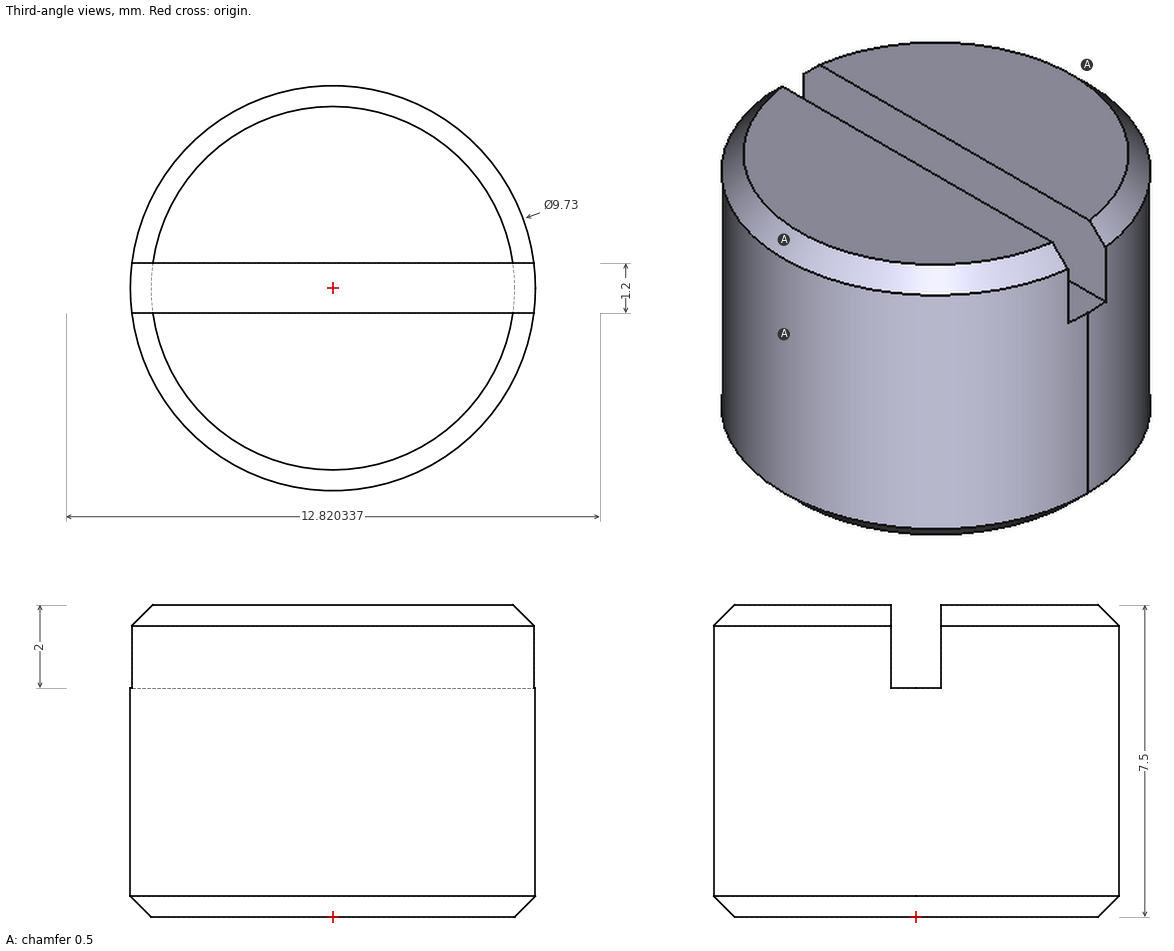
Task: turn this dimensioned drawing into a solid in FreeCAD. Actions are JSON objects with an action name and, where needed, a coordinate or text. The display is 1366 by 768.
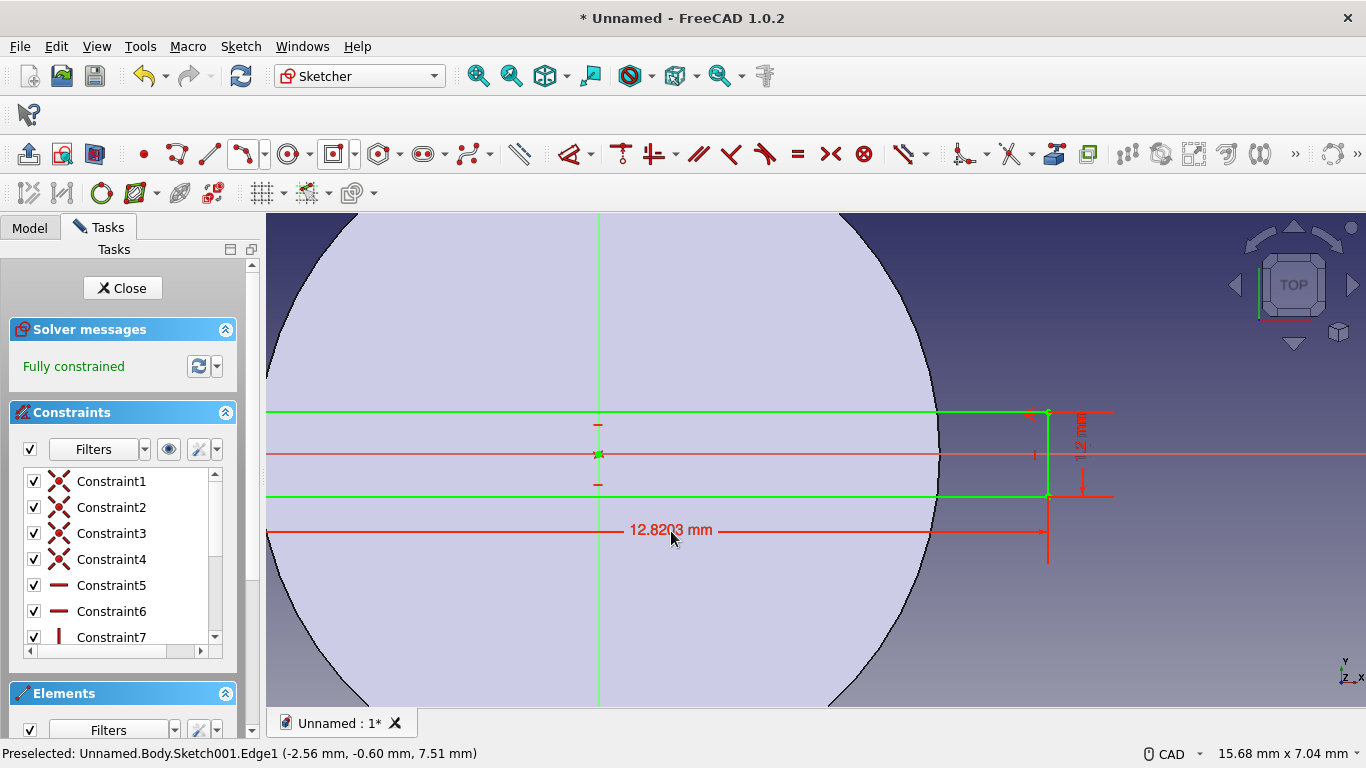
{"action": "left_click", "coordinate": [123, 288]}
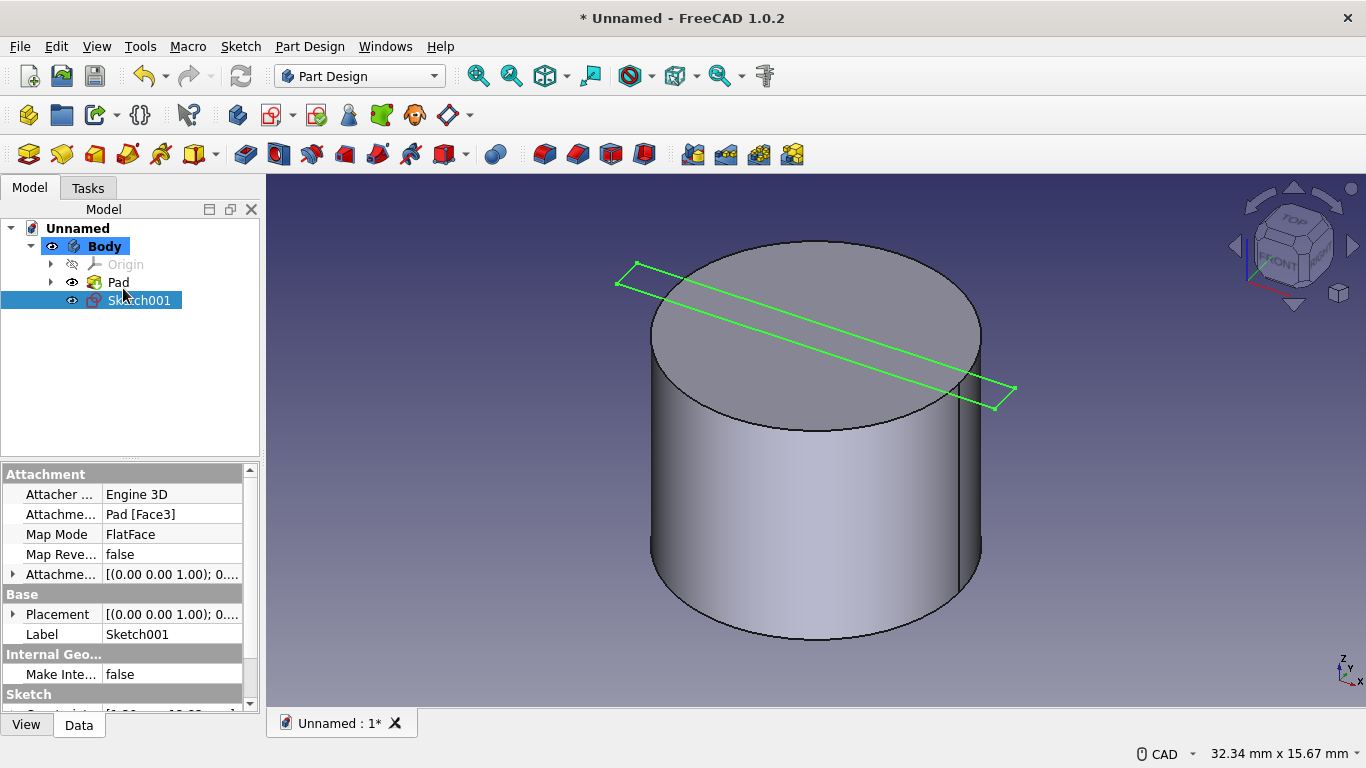
{"action": "left_click", "coordinate": [246, 154]}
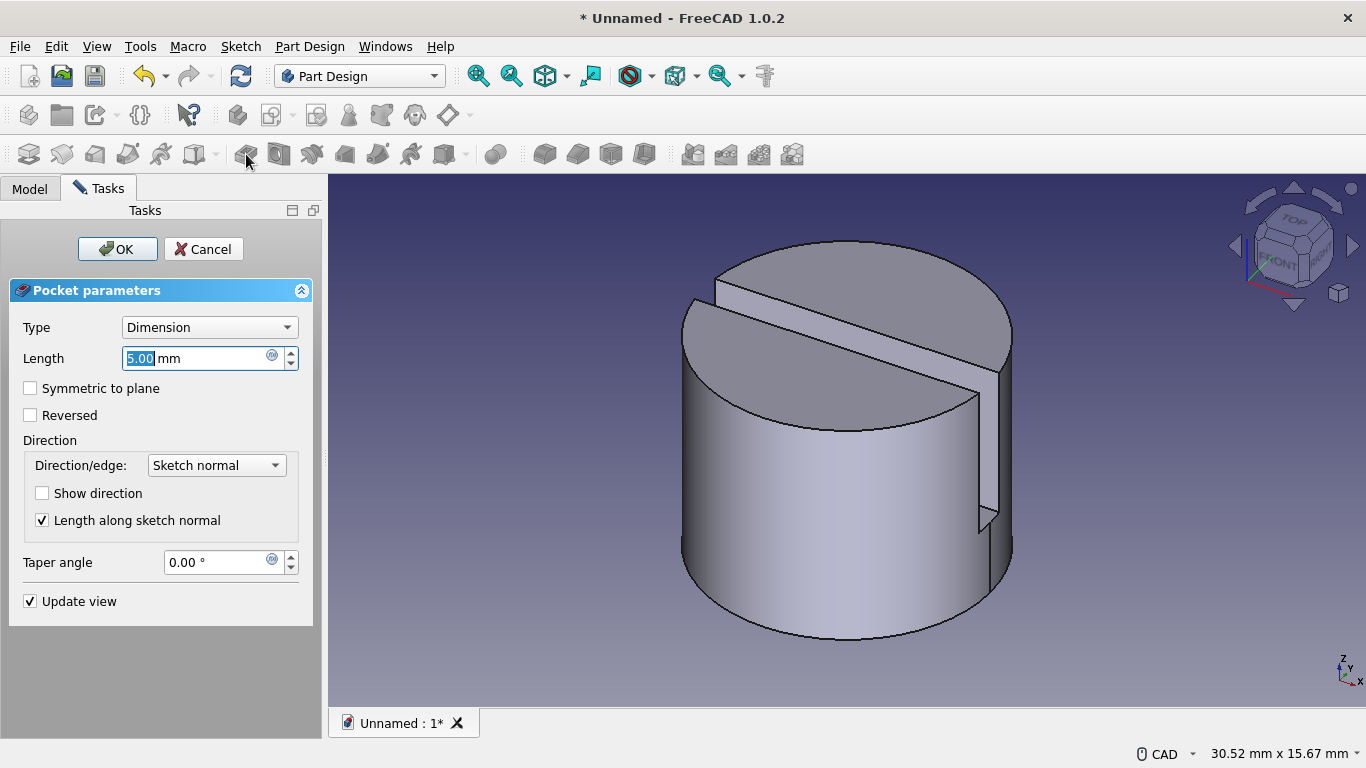
{"action": "type", "text": "2"}
{"action": "key", "text": "Tab"}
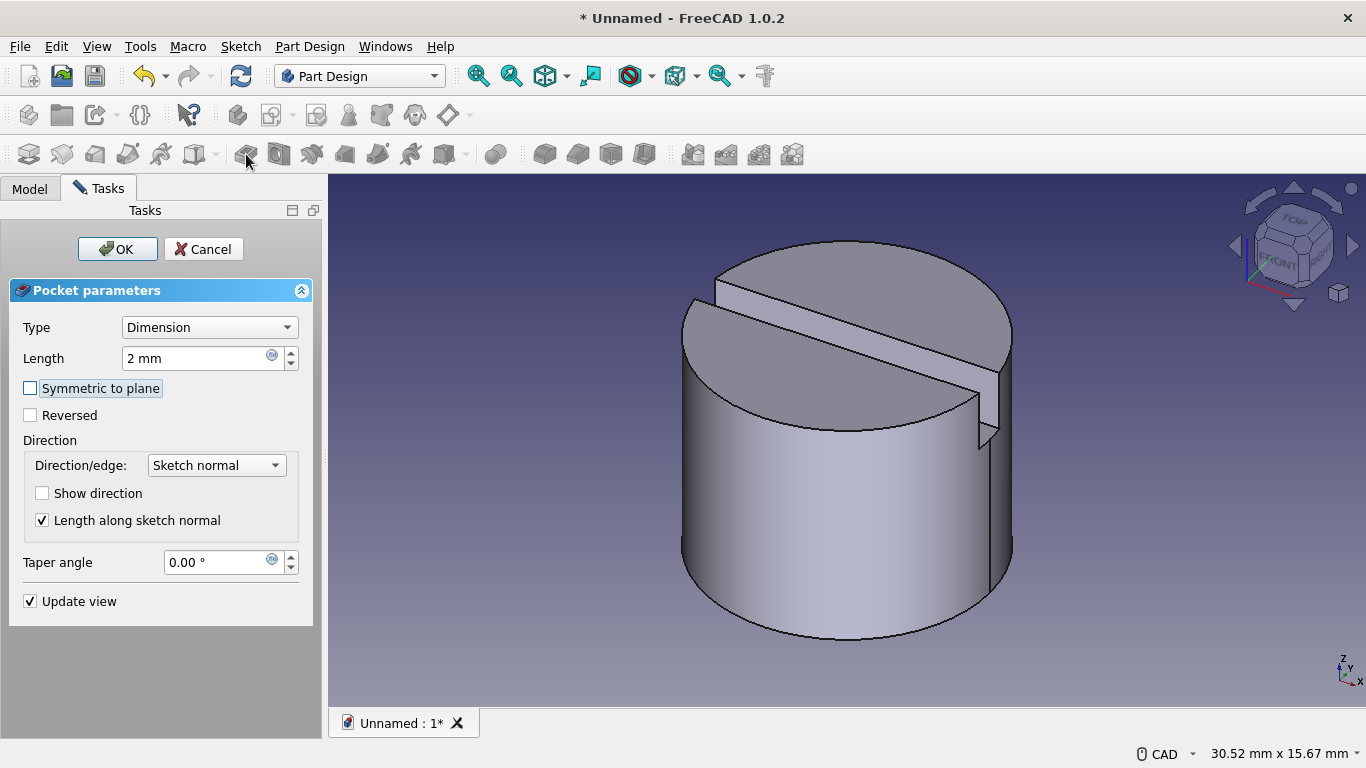
{"action": "left_click", "coordinate": [118, 249]}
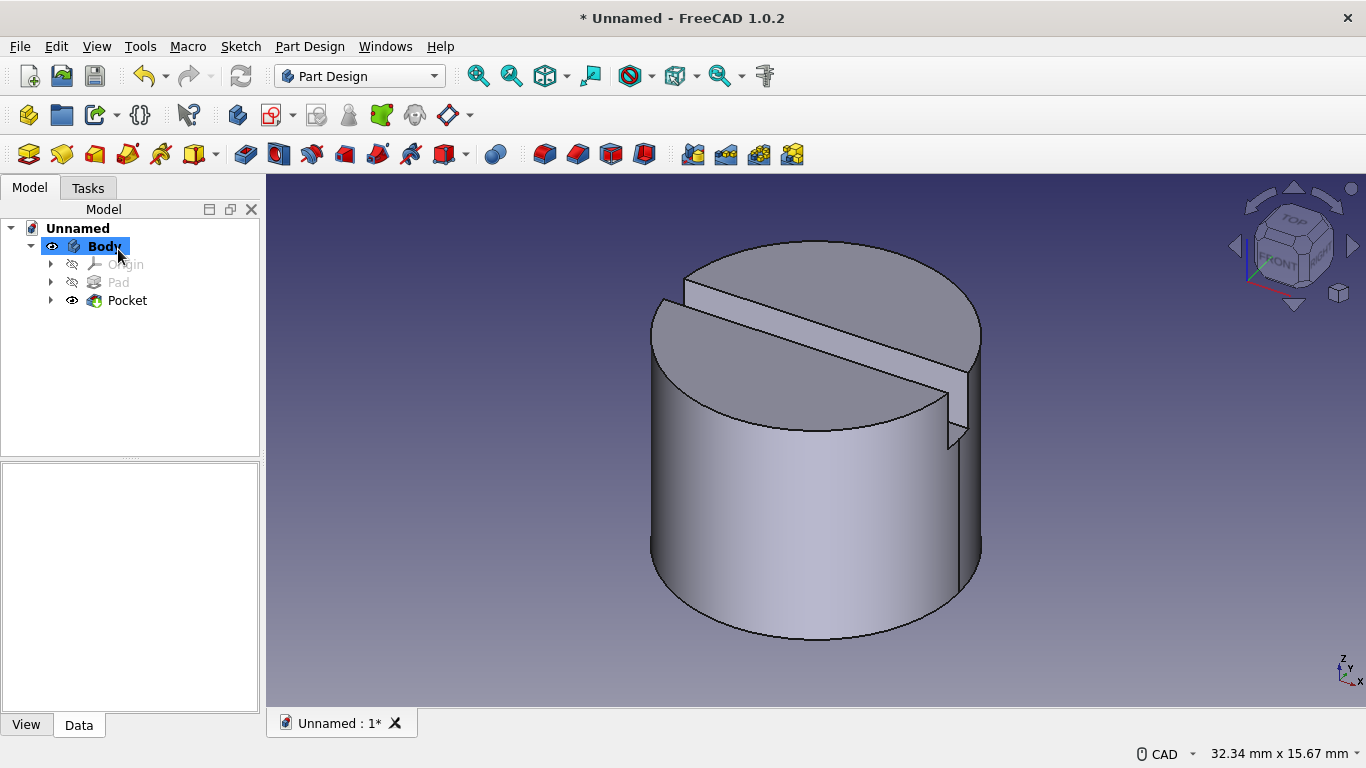
{"action": "left_click", "coordinate": [964, 292]}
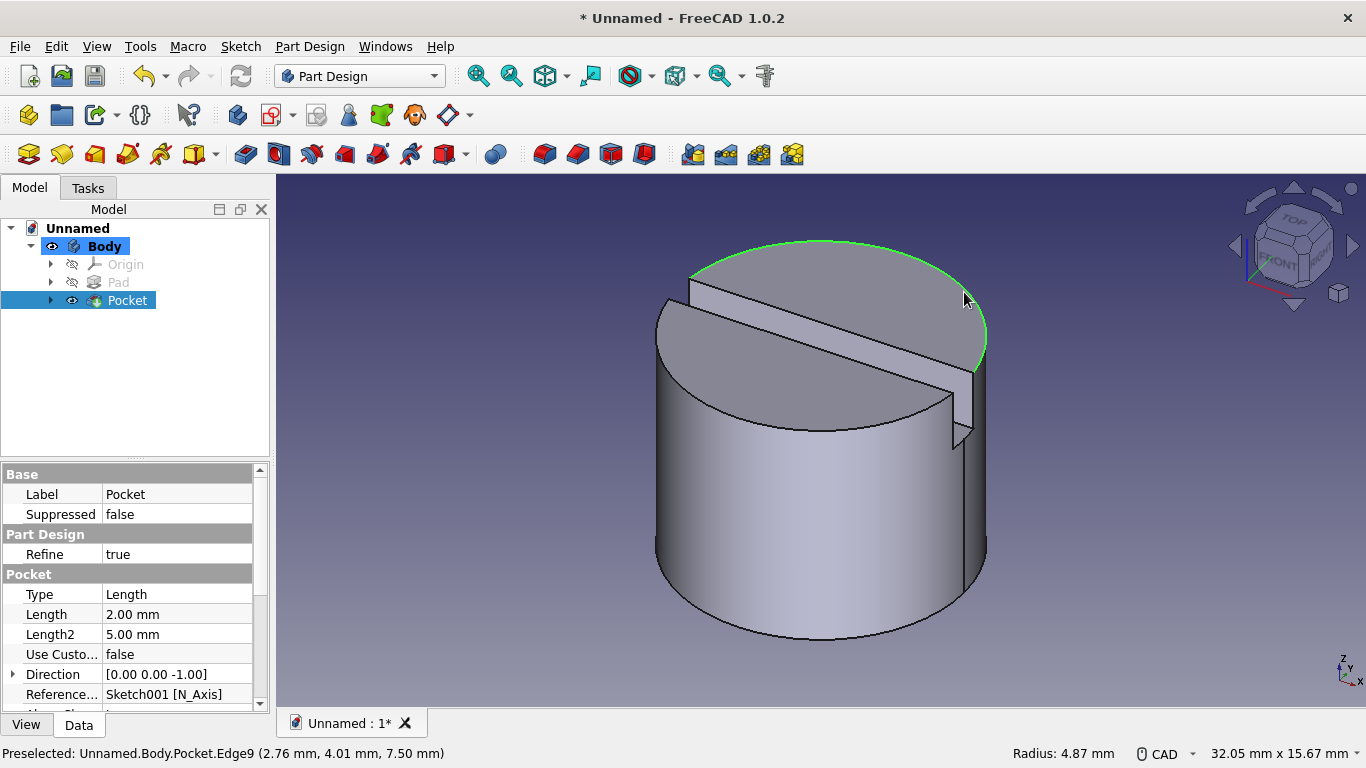
{"action": "left_click", "coordinate": [738, 417], "text": "ctrl"}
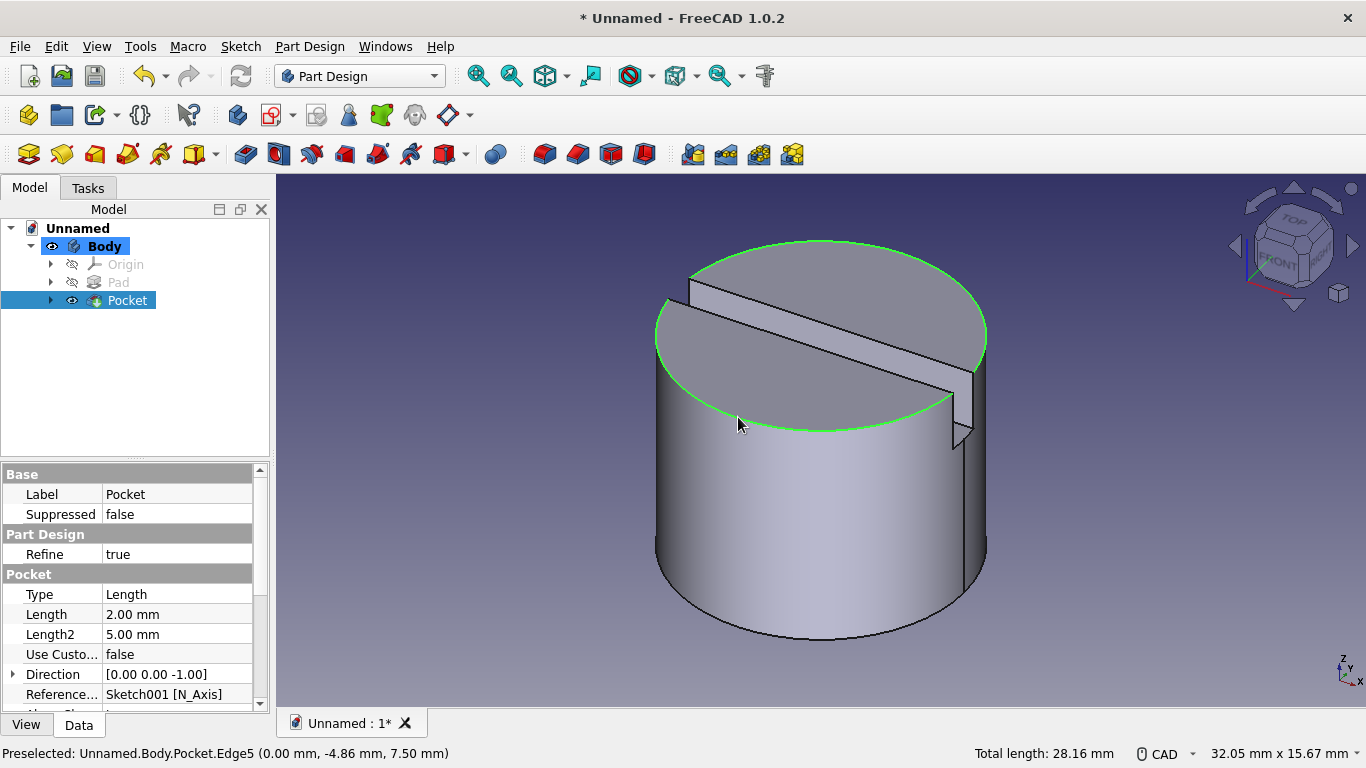
{"action": "key", "text": "0"}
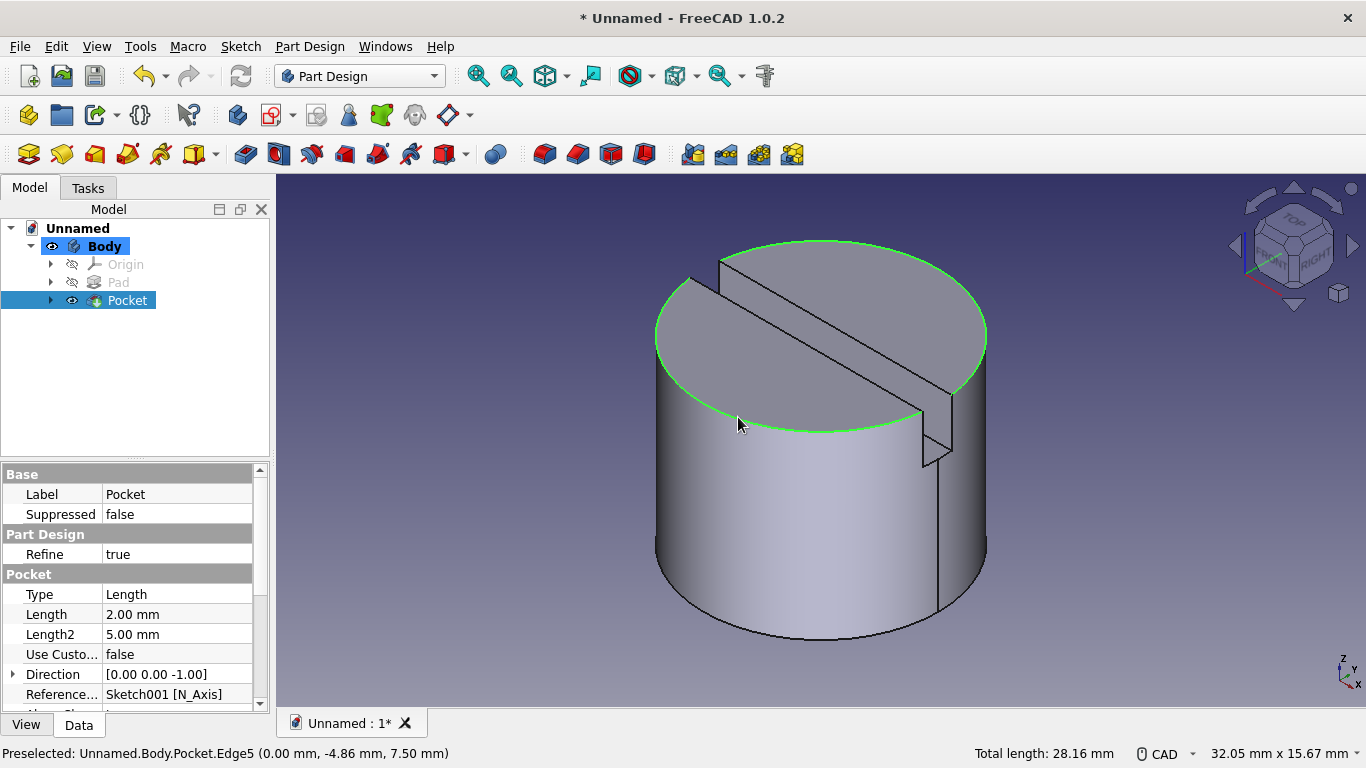
{"action": "key", "text": "2"}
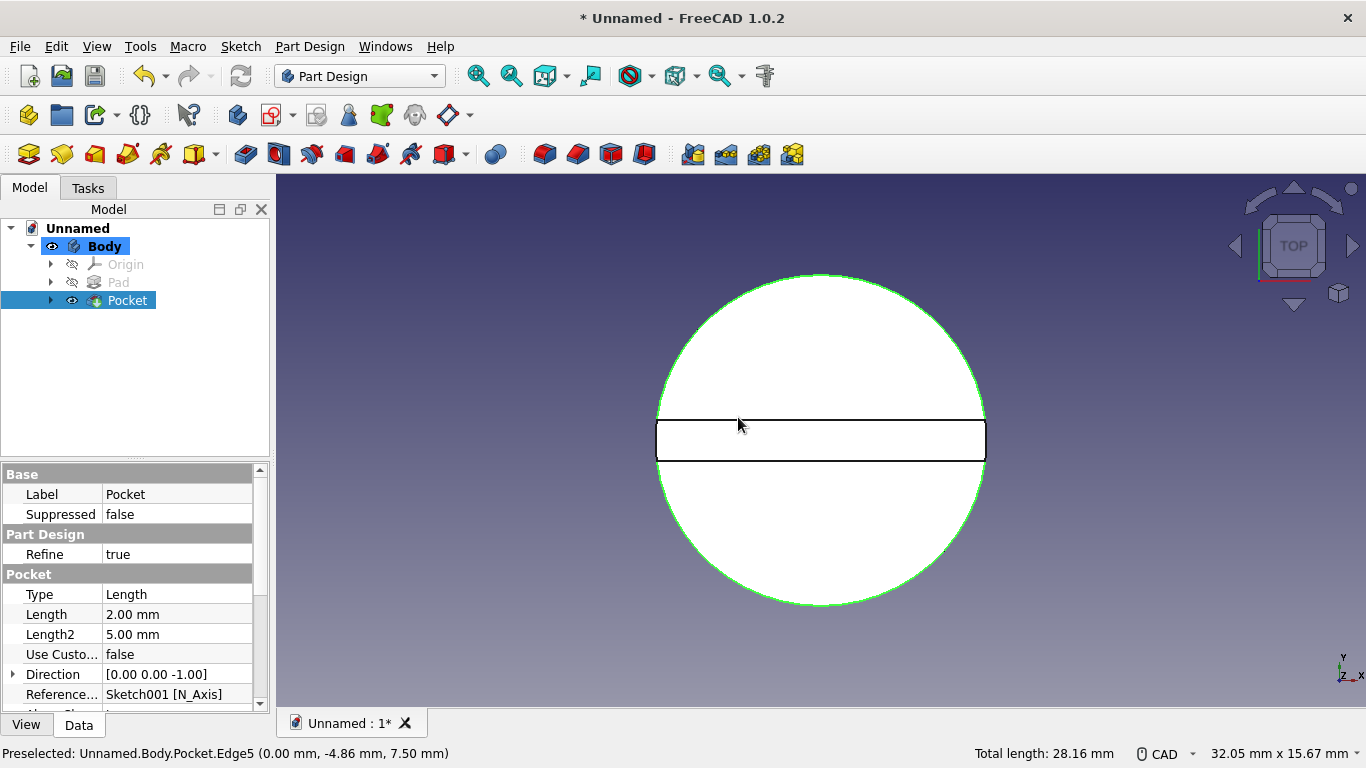
{"action": "key", "text": "1"}